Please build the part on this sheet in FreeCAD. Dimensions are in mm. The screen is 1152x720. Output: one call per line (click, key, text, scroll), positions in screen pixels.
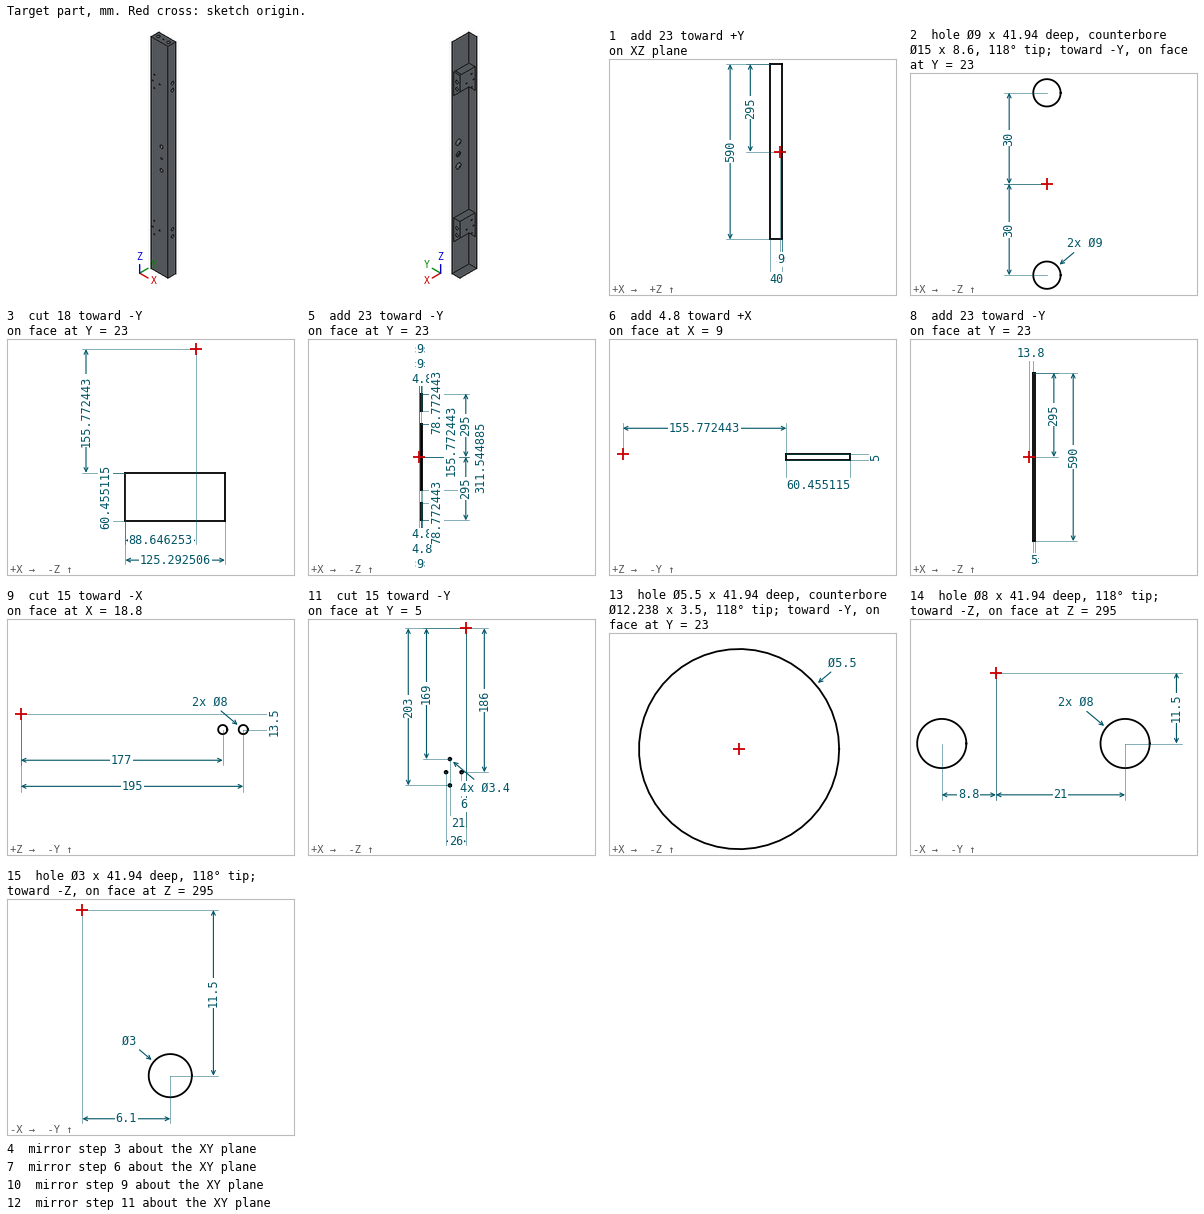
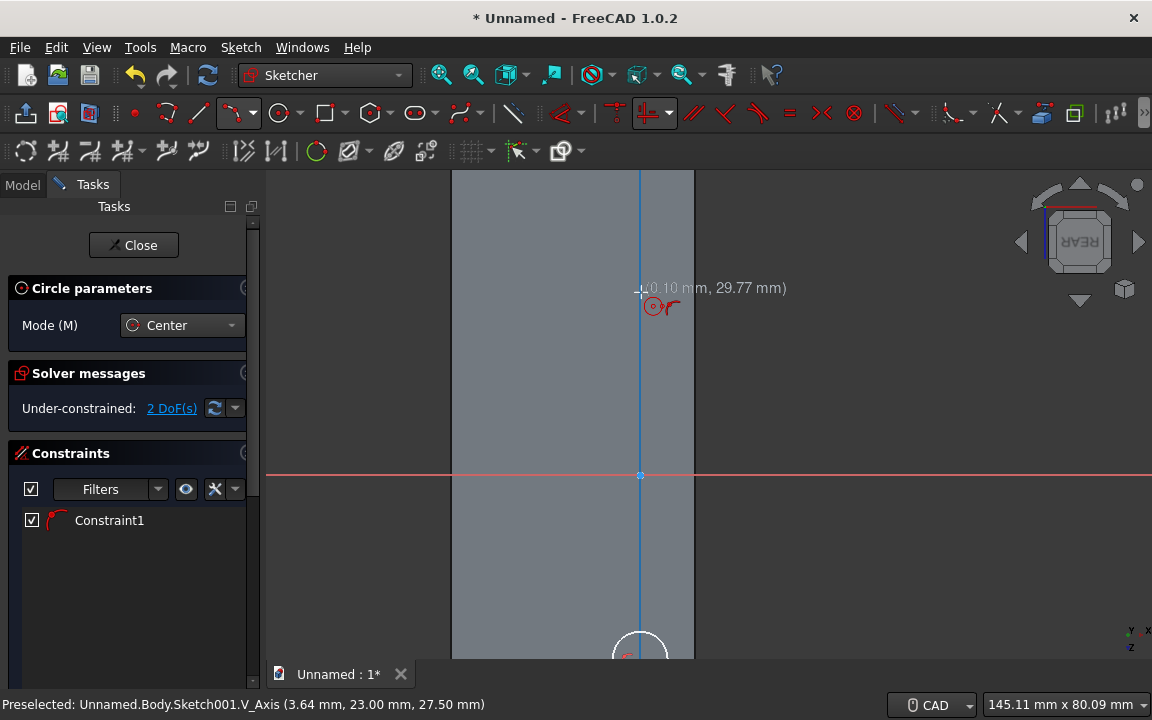
click(640, 292)
click(660, 273)
key(Escape)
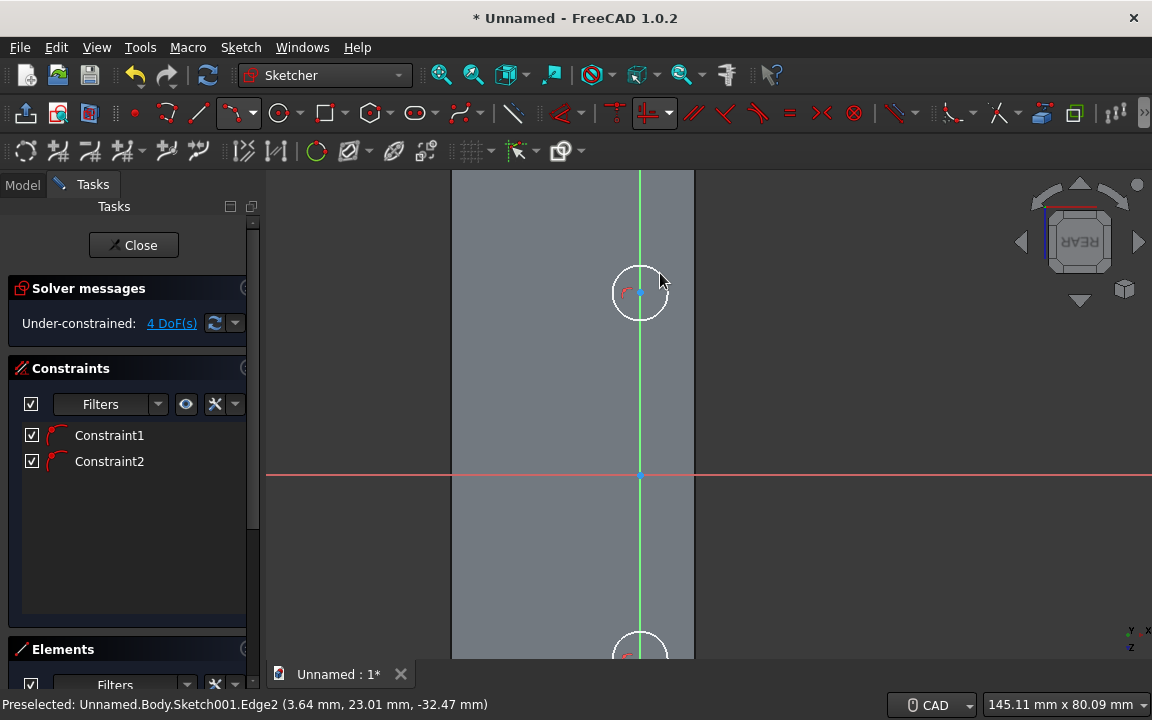
scroll(641, 291, down, 2)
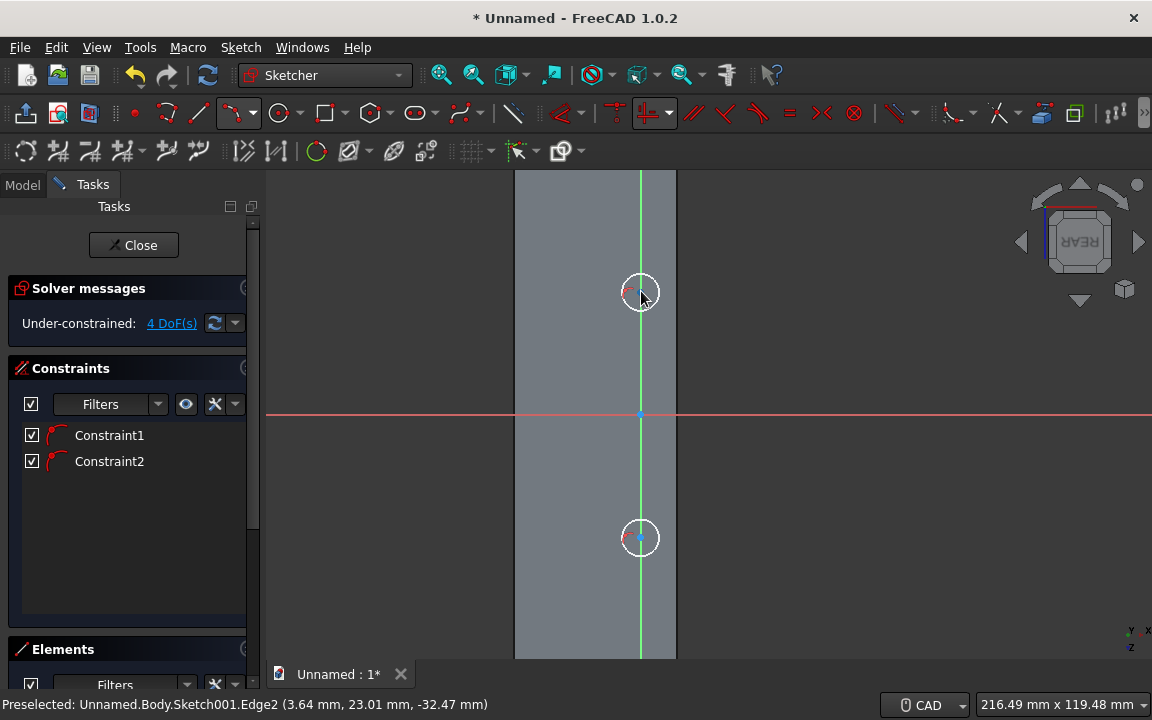
click(654, 525)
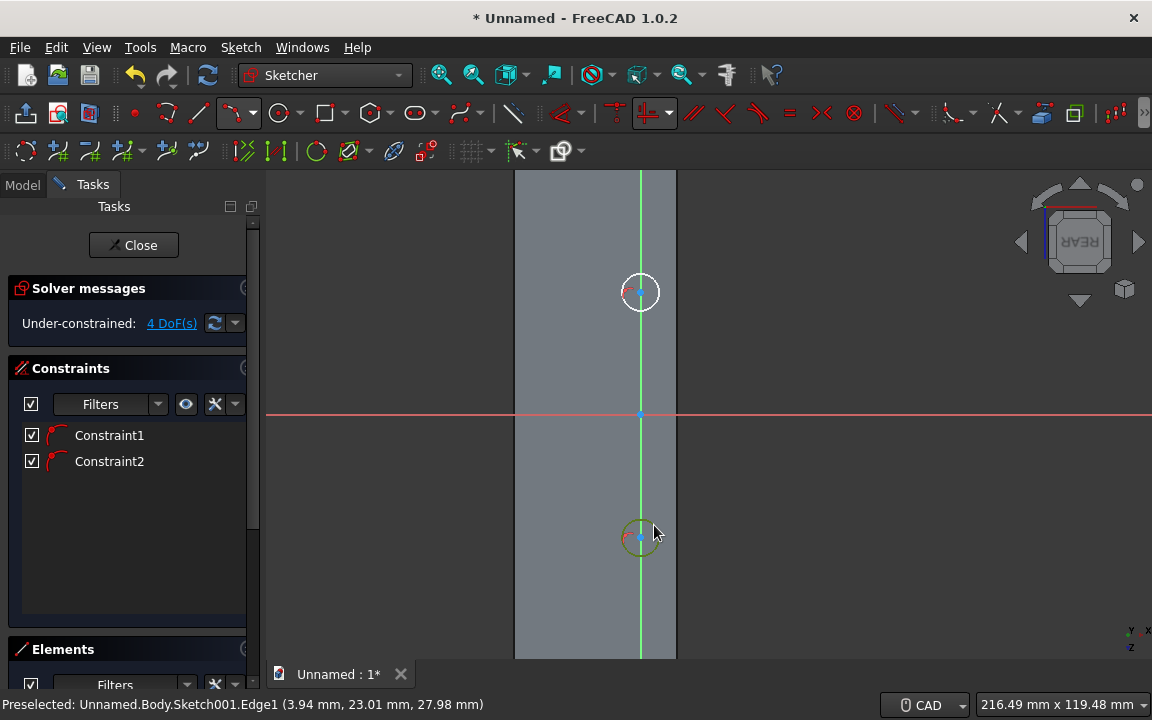
click(654, 279)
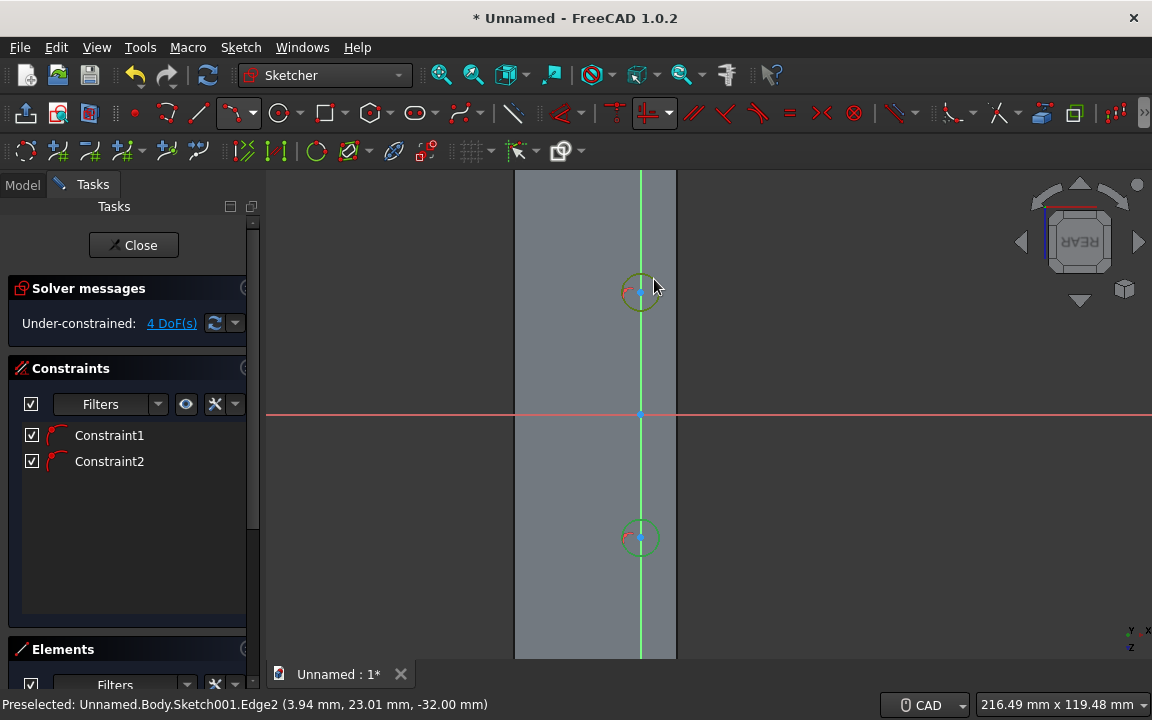
click(790, 114)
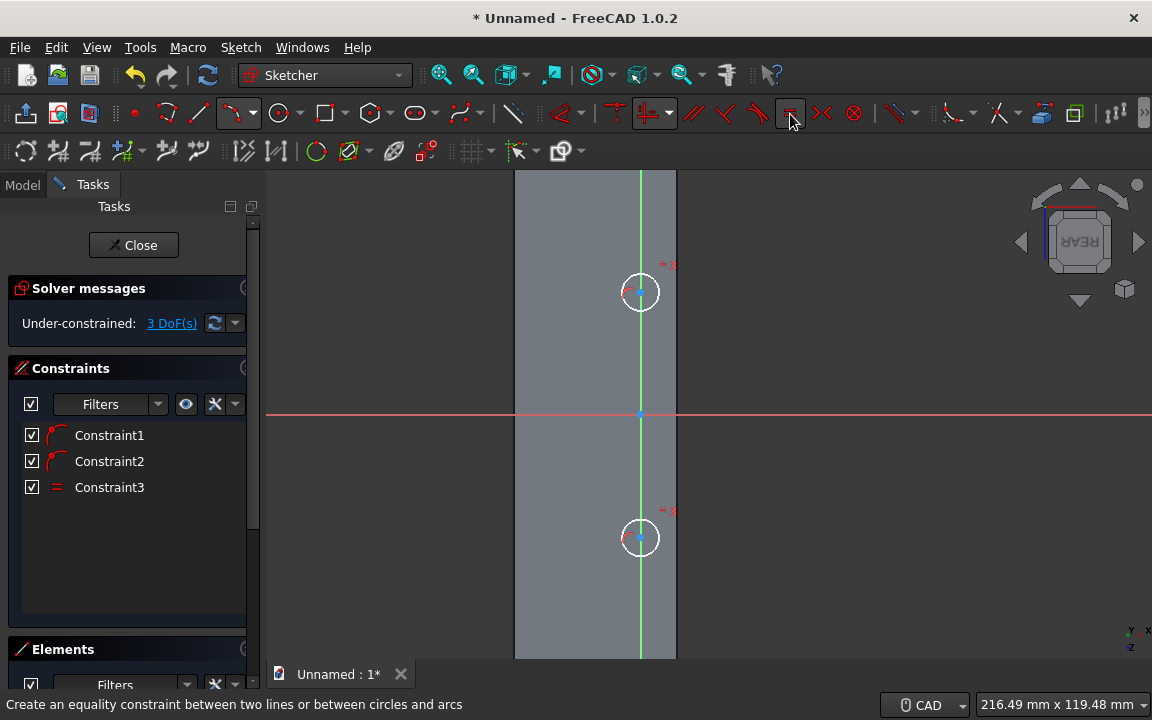
click(560, 114)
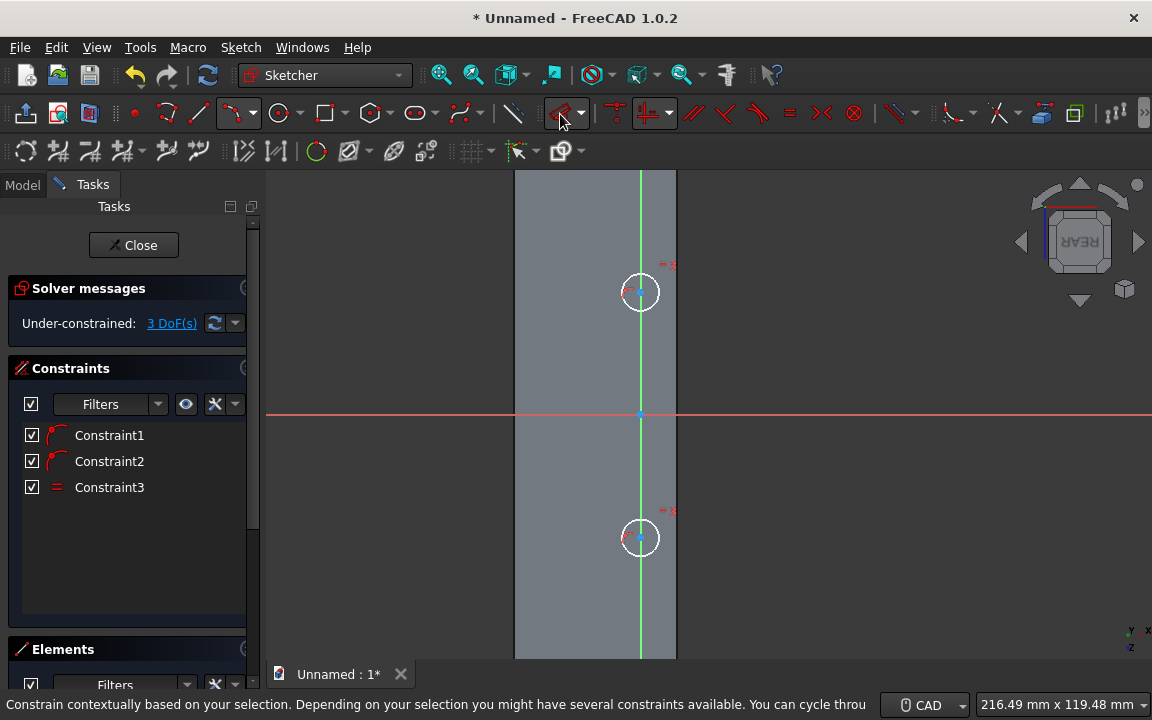
click(654, 525)
click(677, 503)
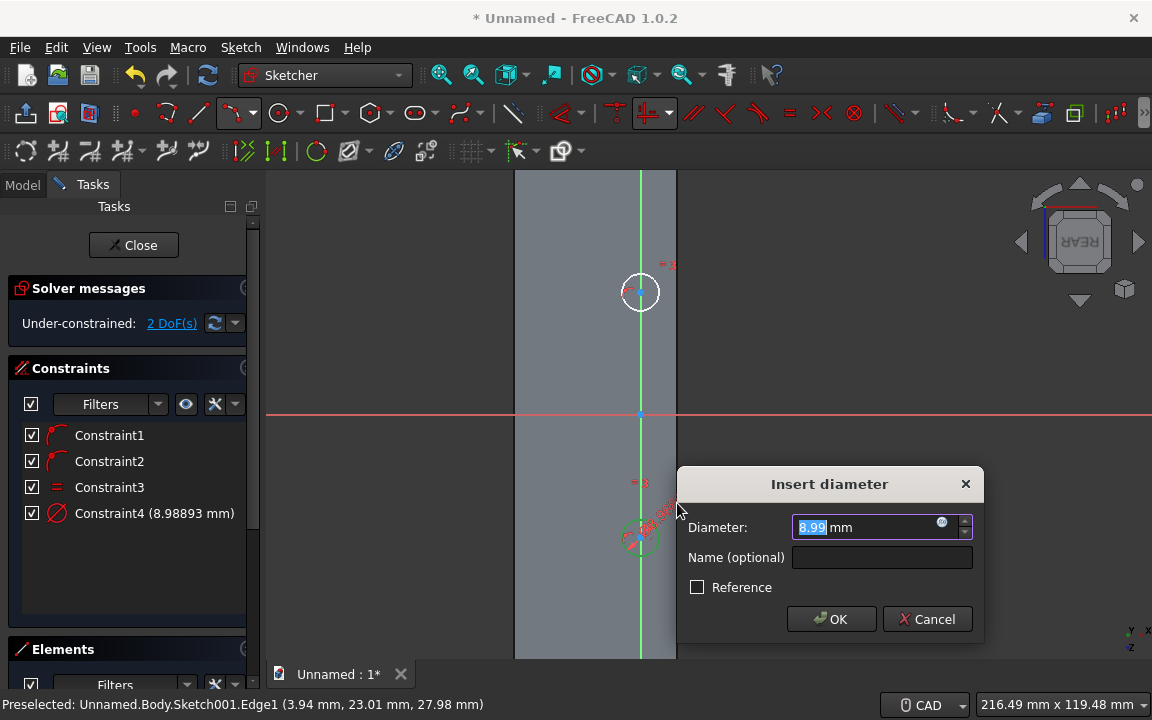
text(9)
key(Return)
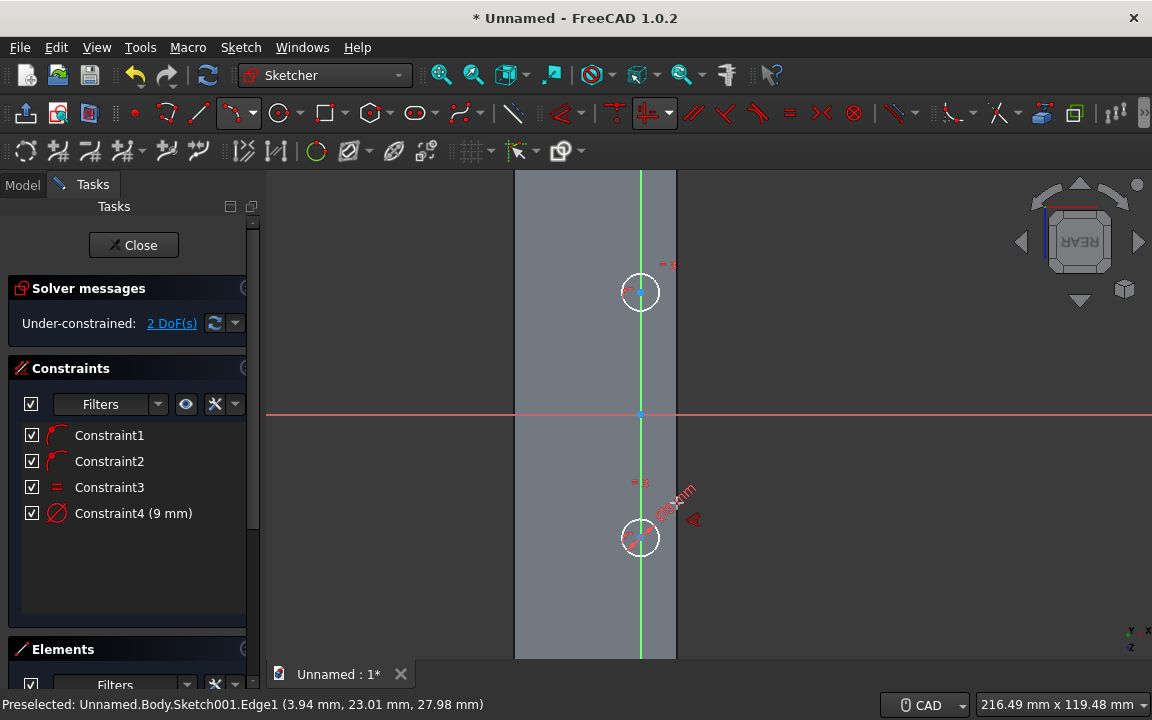
click(641, 538)
click(675, 476)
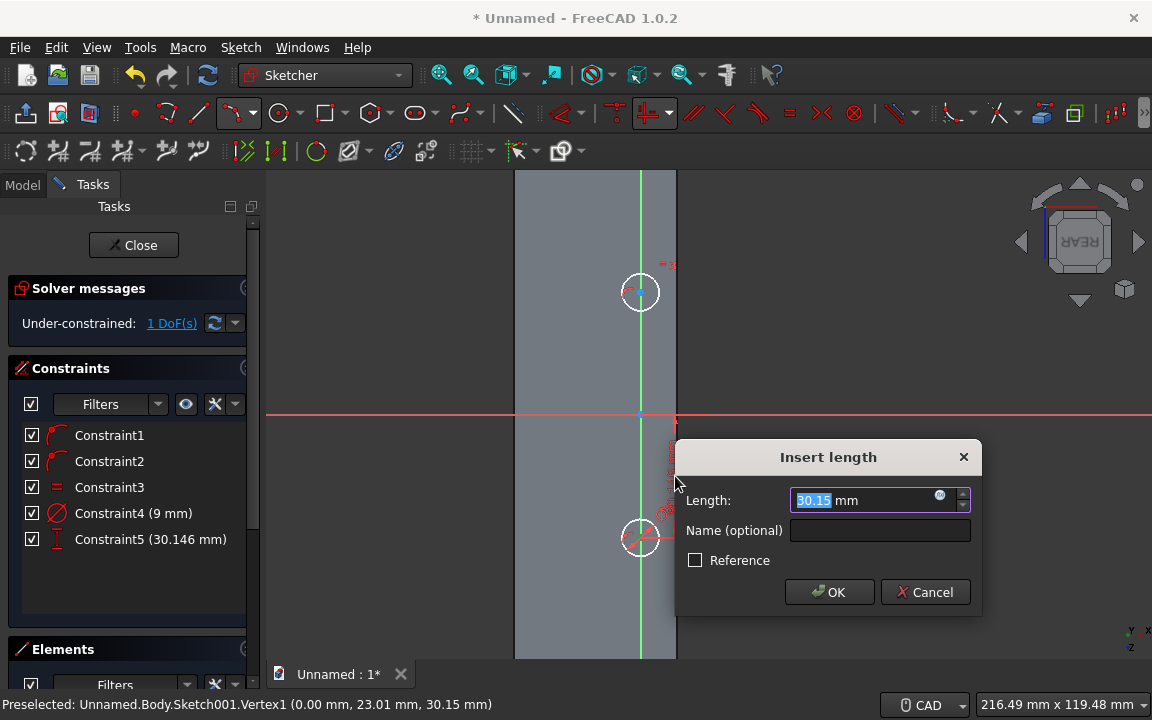
text(30)
key(Return)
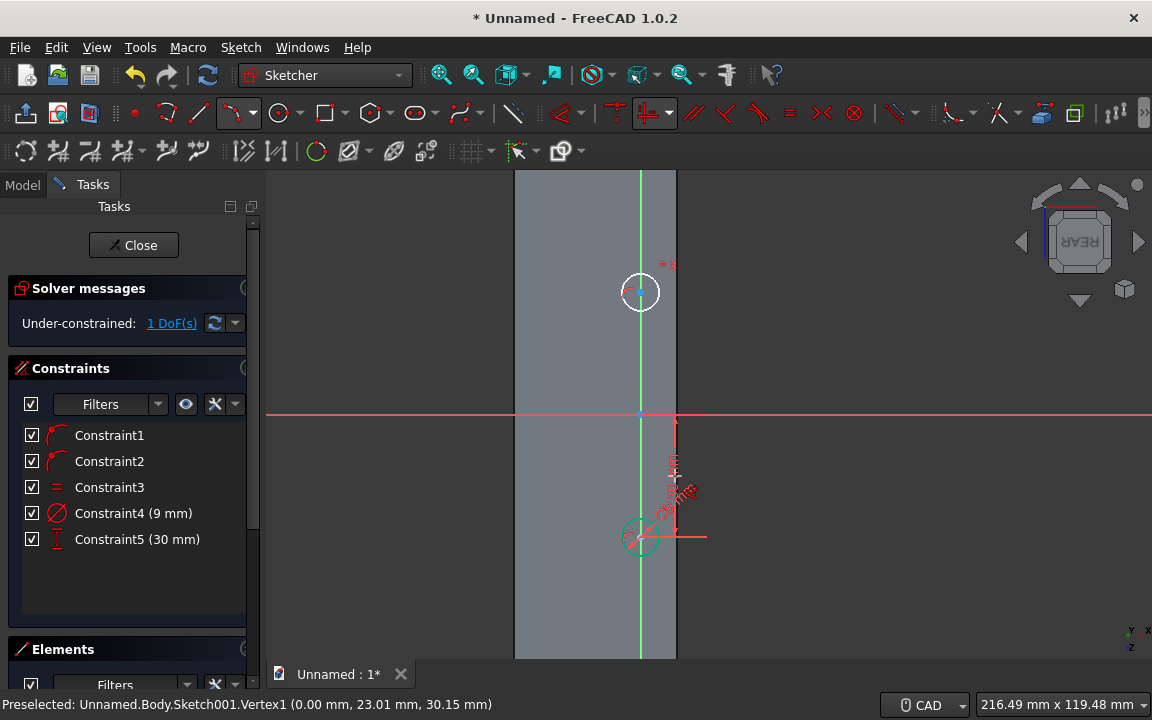
click(641, 292)
click(675, 353)